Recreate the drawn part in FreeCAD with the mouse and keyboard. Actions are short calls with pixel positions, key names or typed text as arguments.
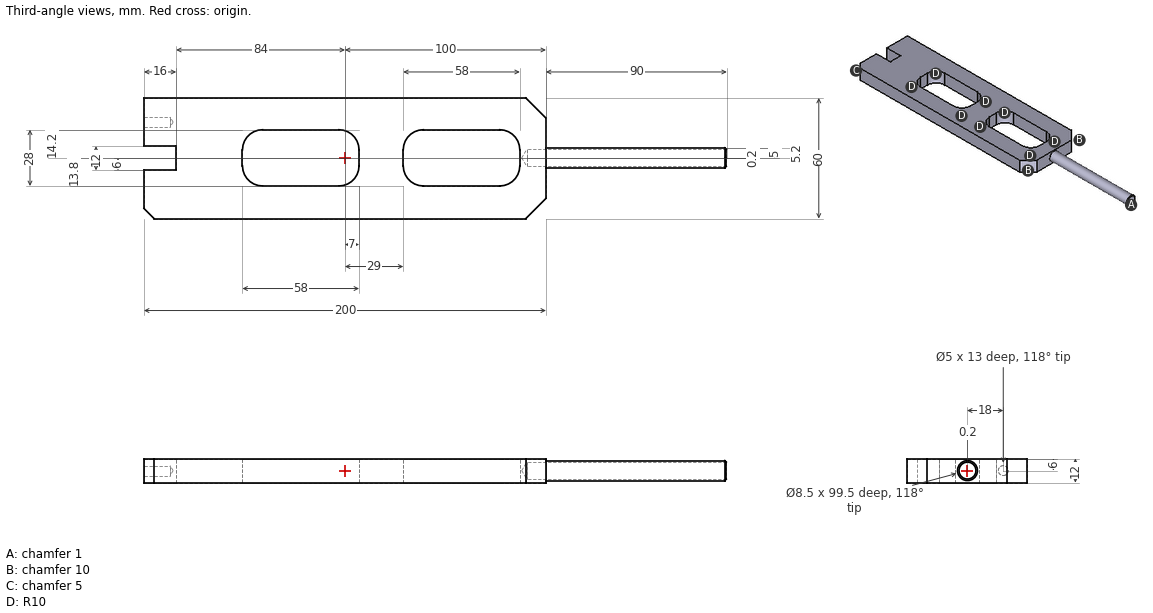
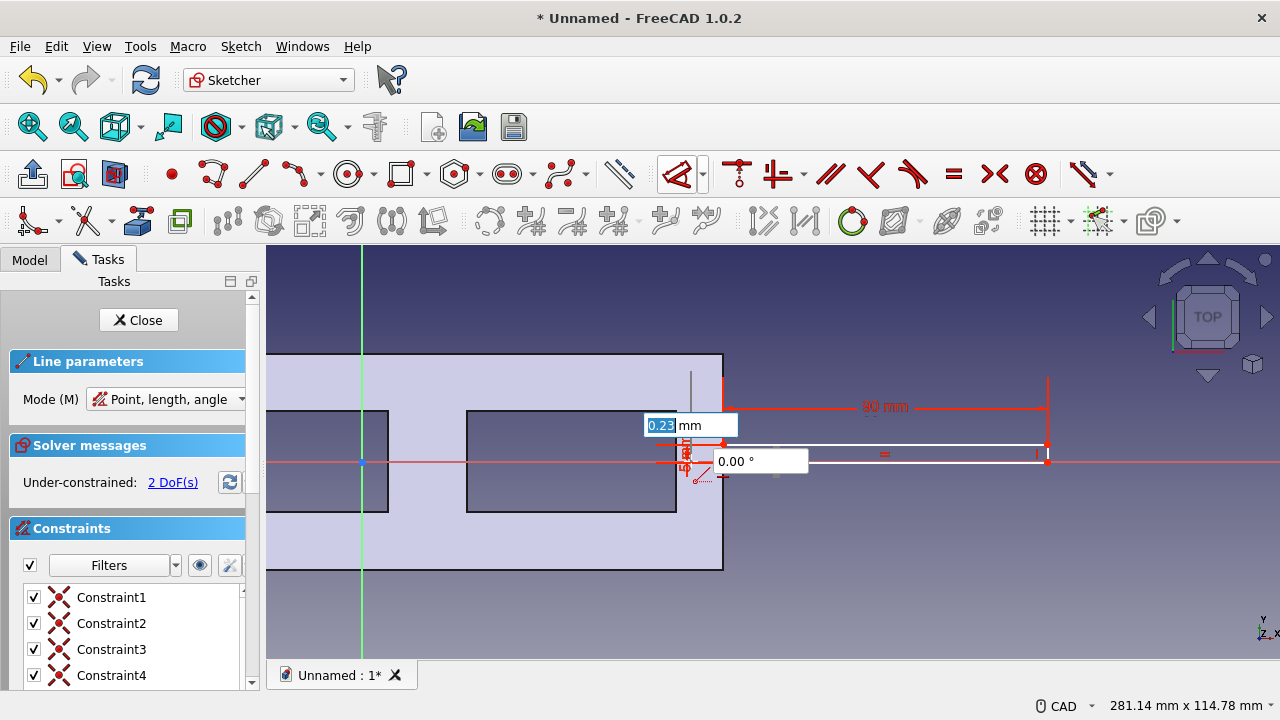
scroll(593, 461, up, 16)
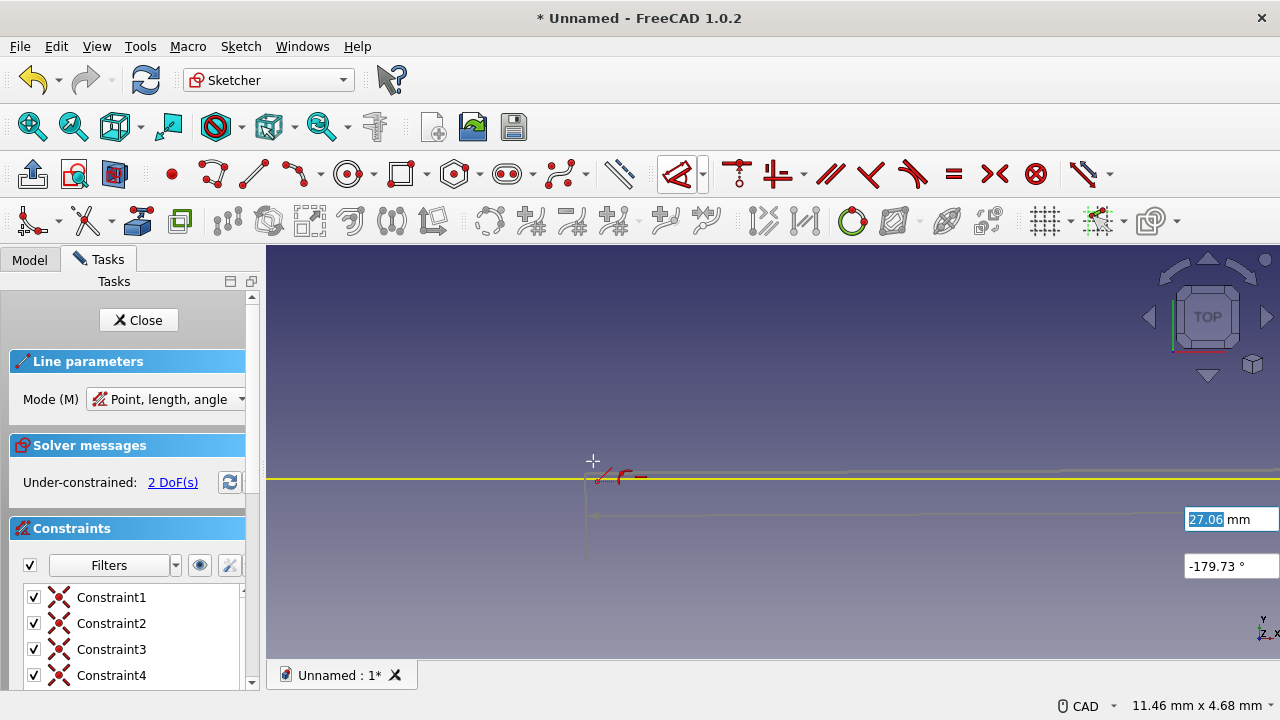
click(590, 461)
key(Escape)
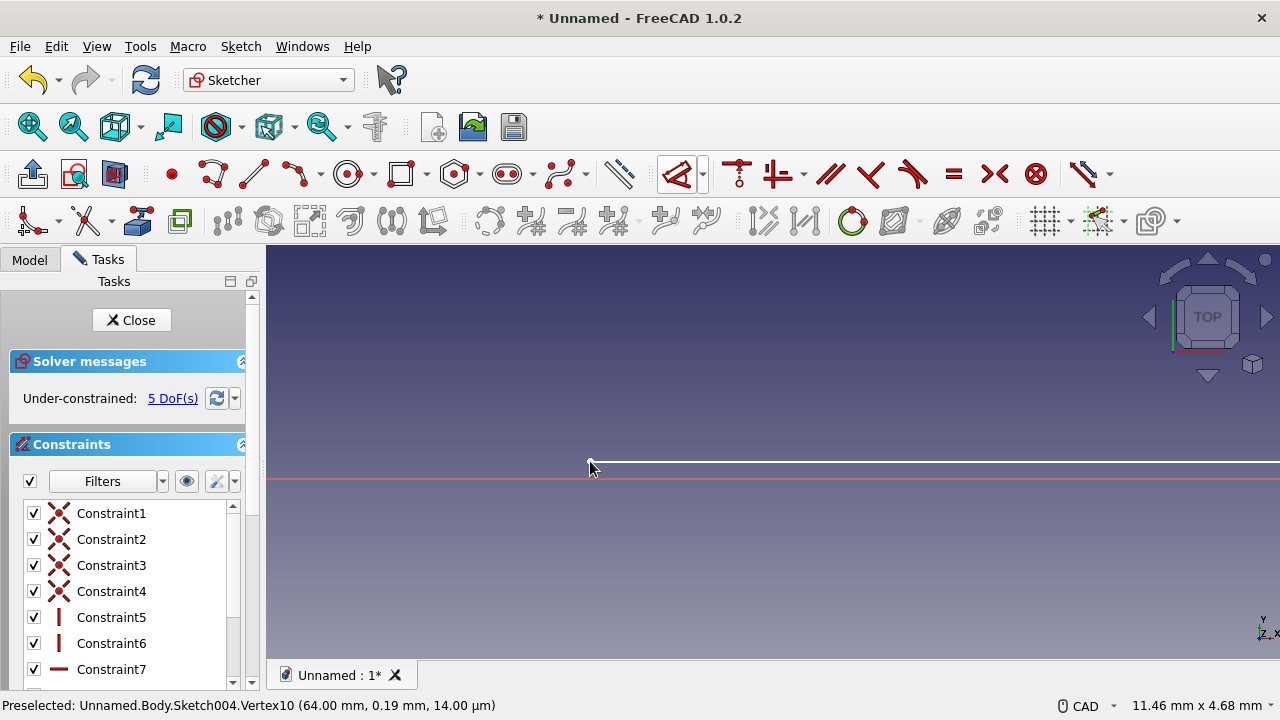
click(1068, 462)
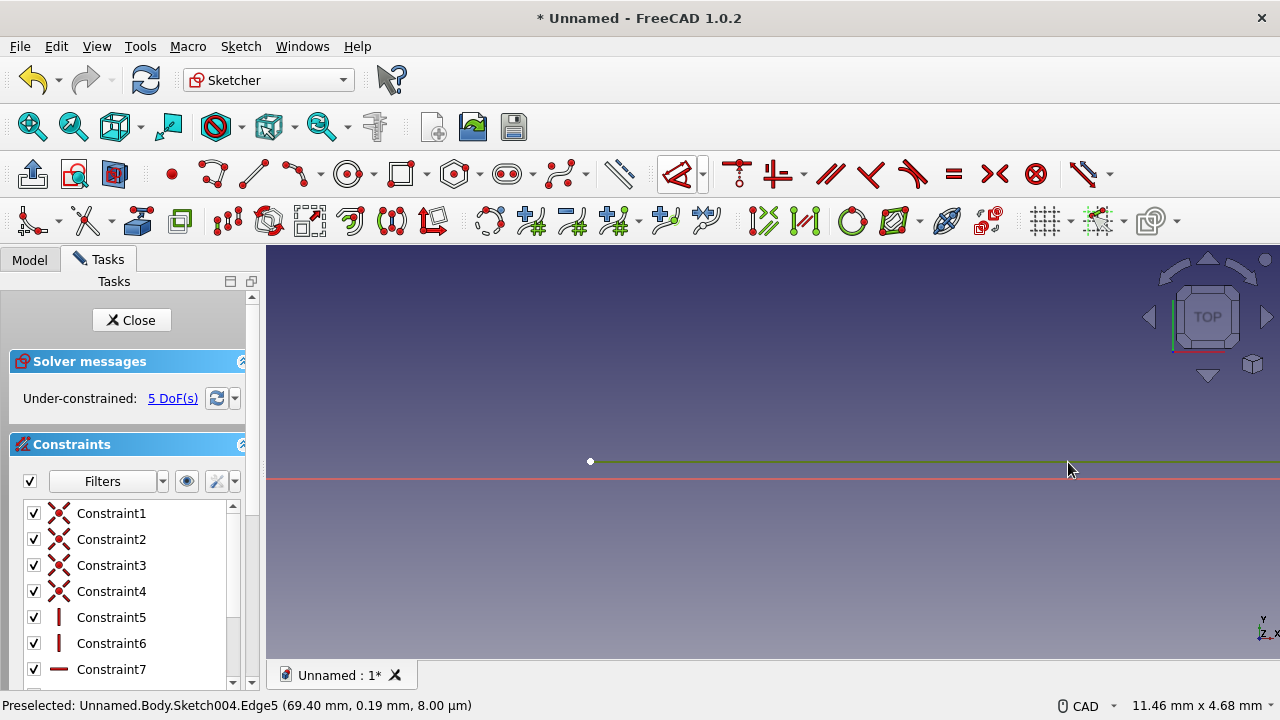
key(g)
key(n)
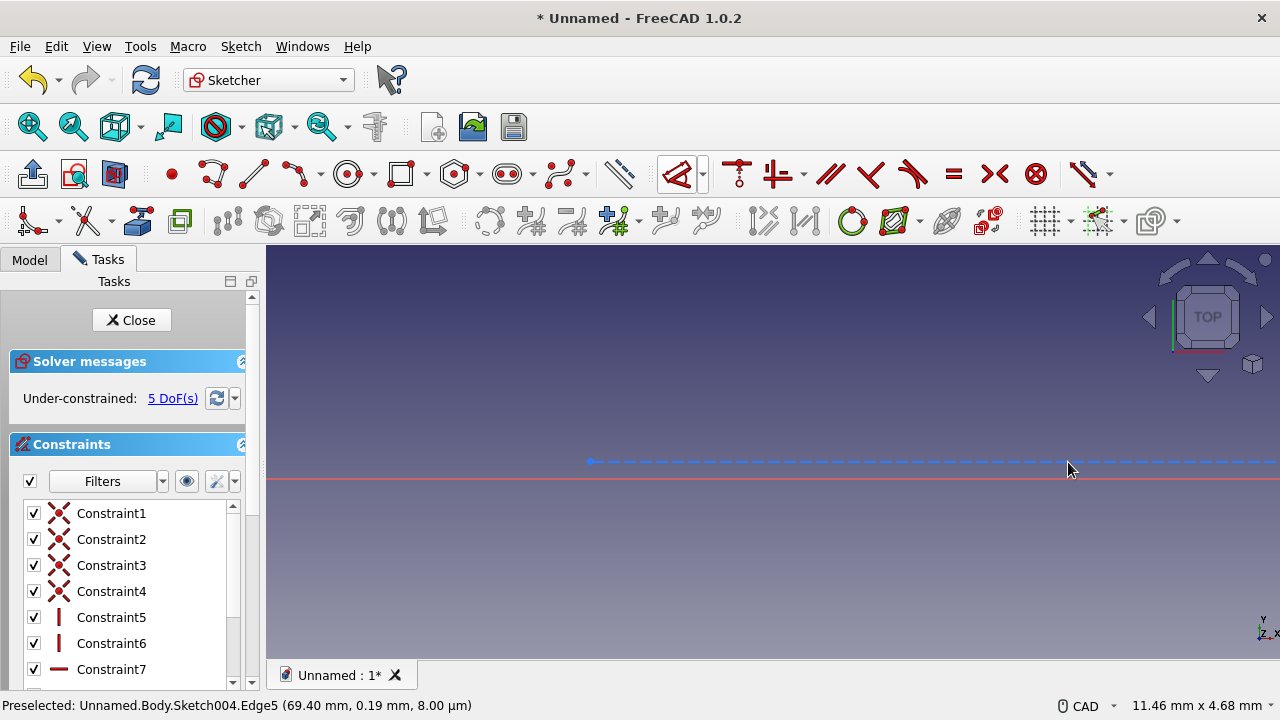
scroll(593, 461, down, 16)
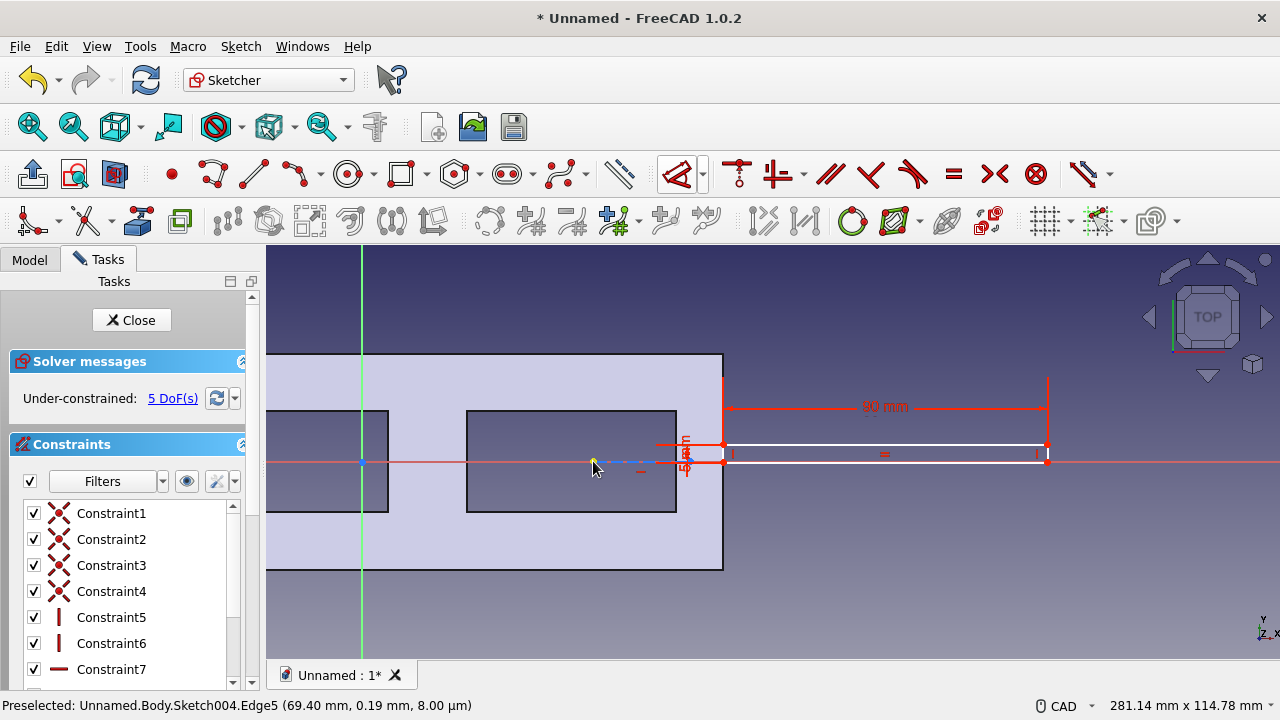
click(723, 445)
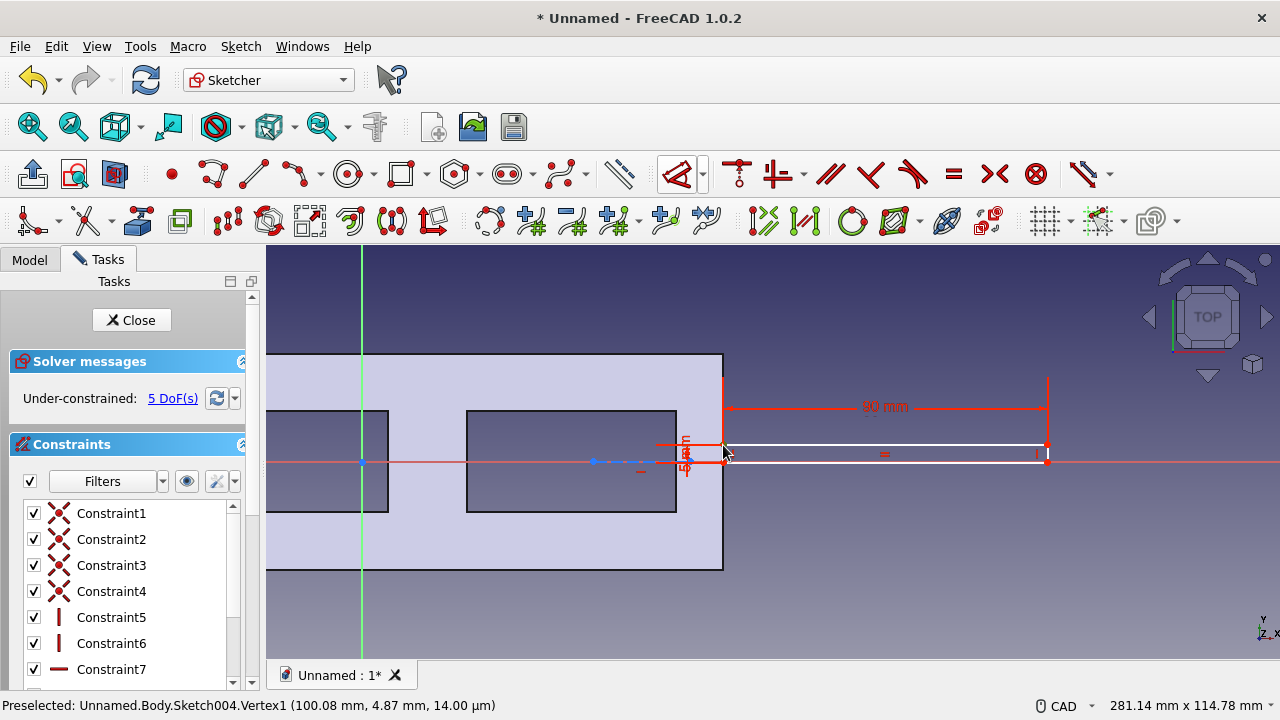
click(702, 174)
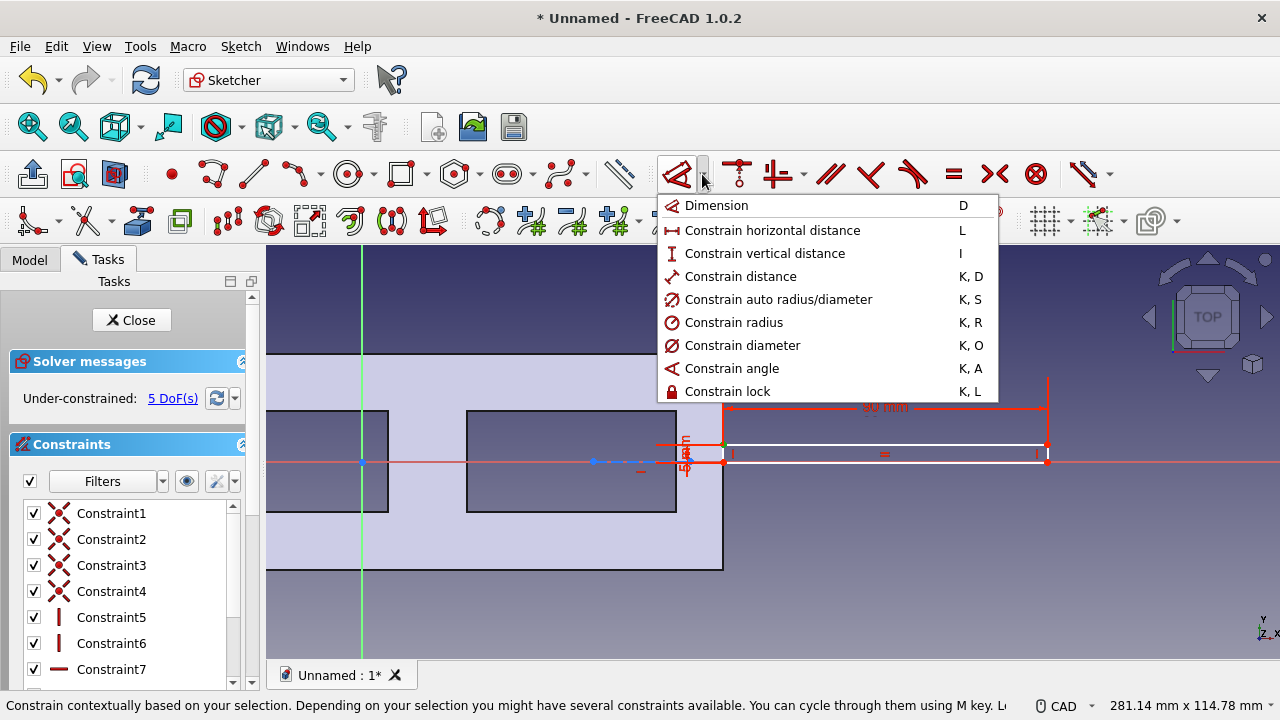
click(828, 230)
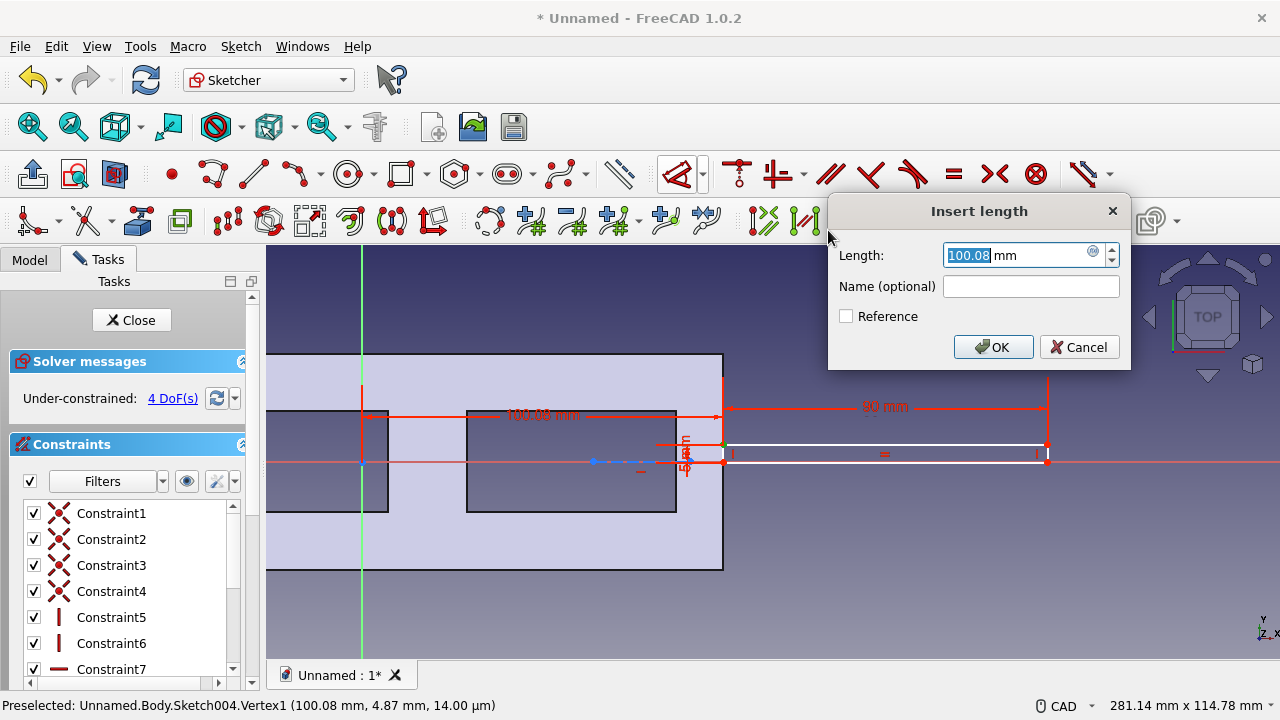
text(100)
key(Return)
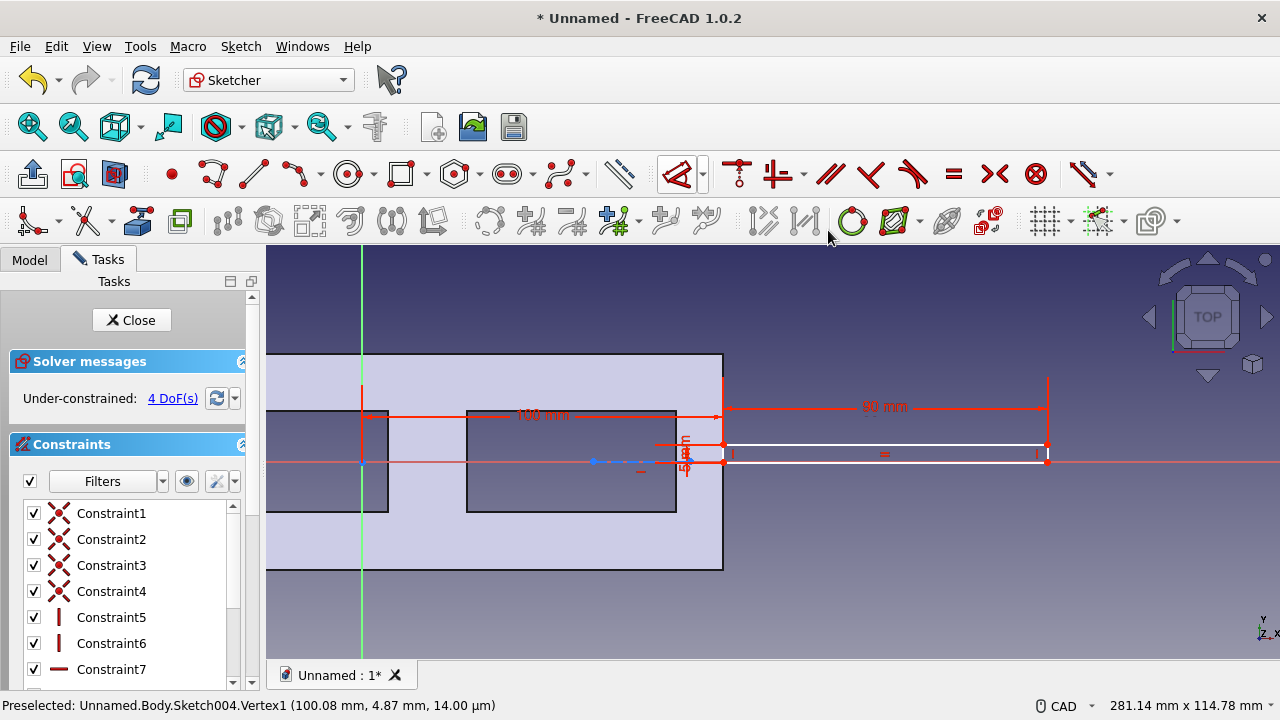
scroll(723, 445, up, 4)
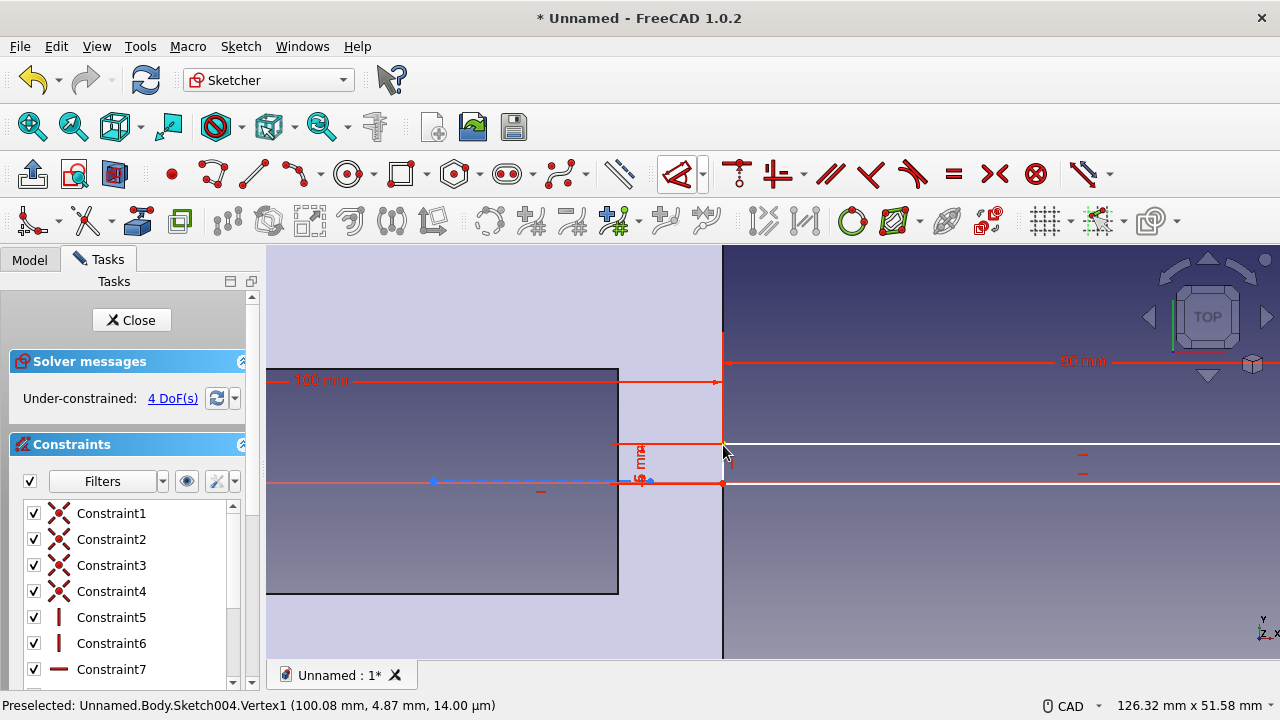
click(723, 444)